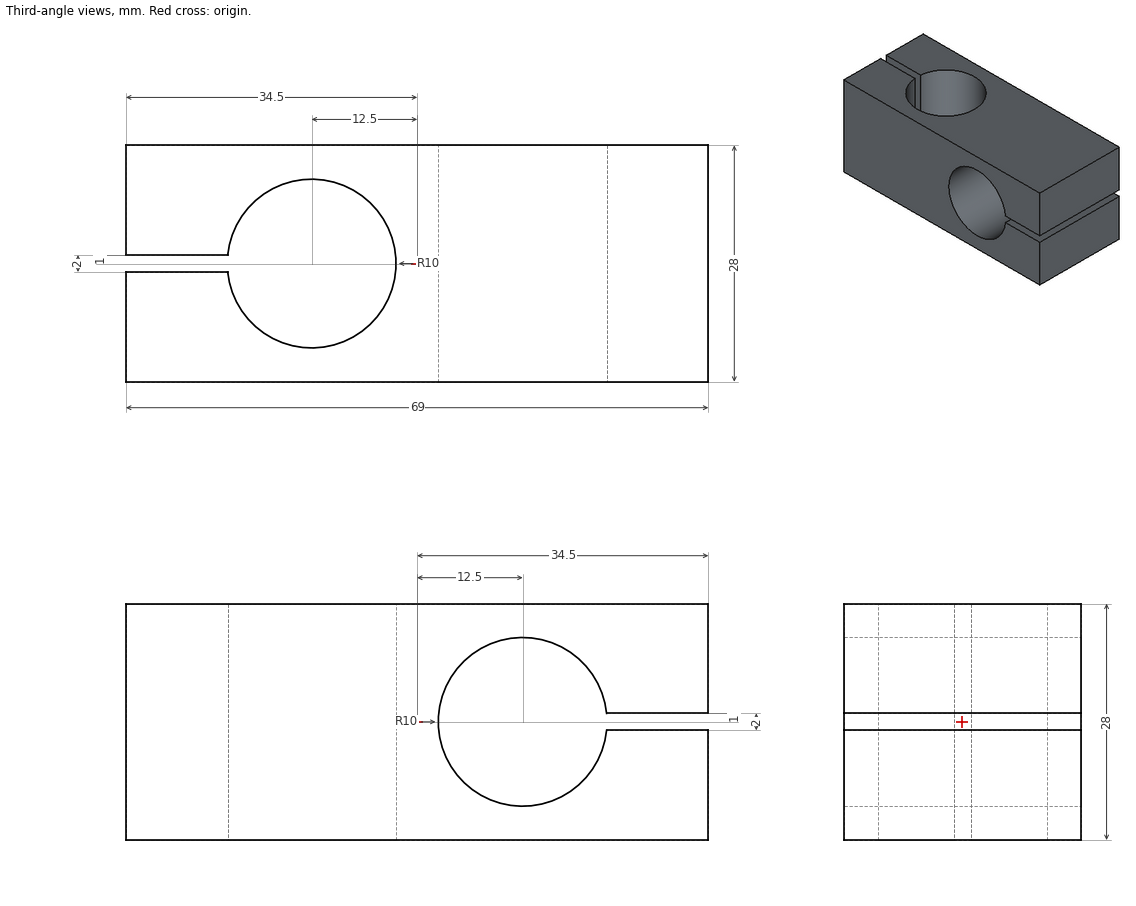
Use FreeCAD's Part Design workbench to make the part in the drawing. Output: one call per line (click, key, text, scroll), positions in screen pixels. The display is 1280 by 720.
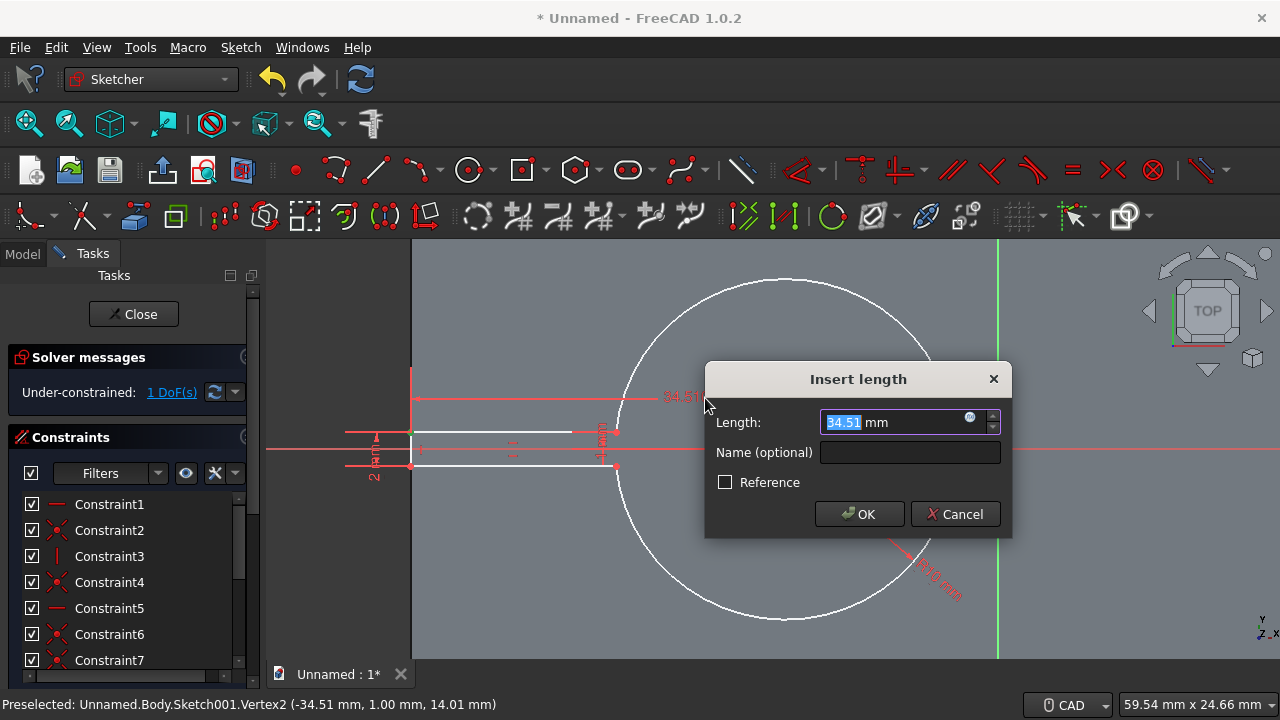
text(34.5)
key(Return)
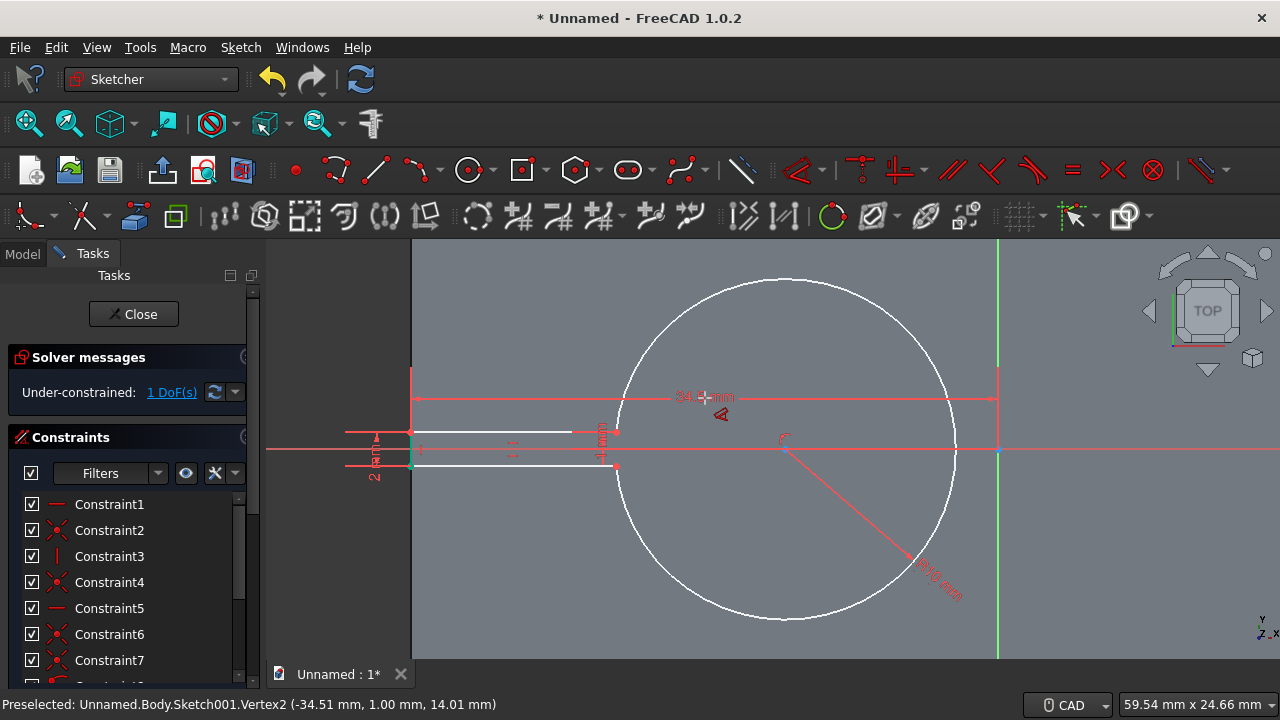
click(786, 449)
click(892, 483)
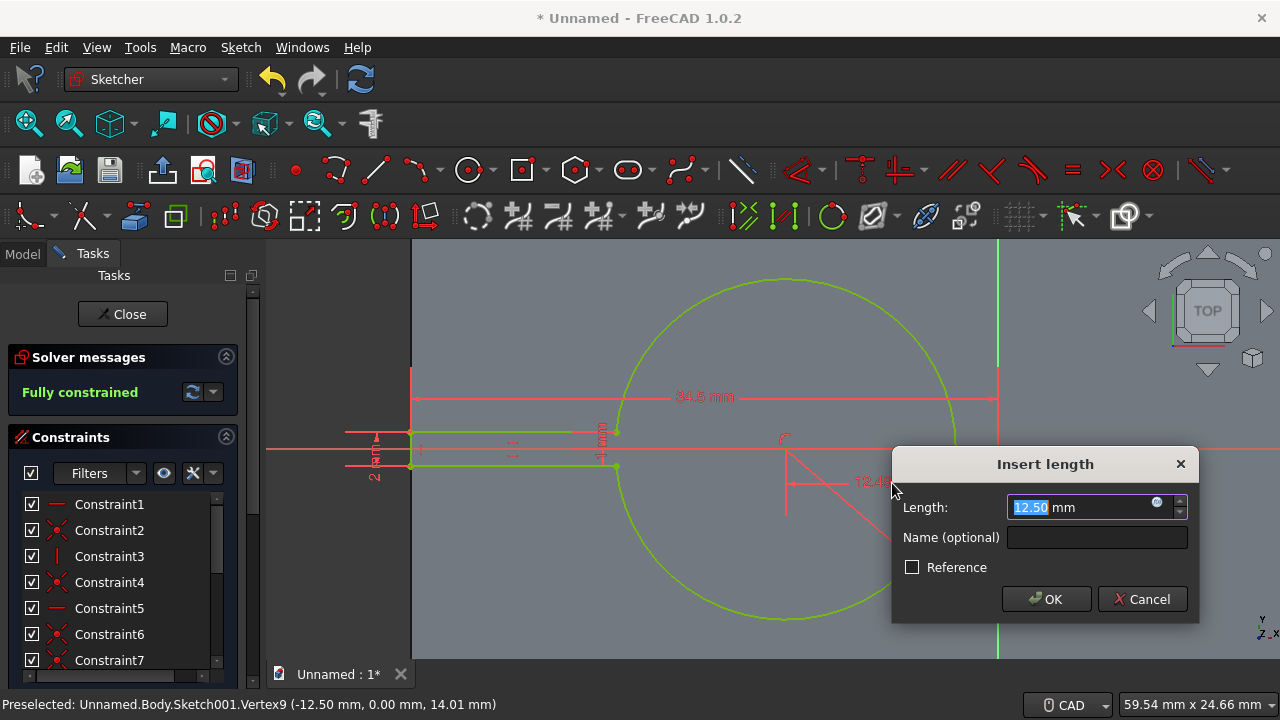
text(12.5)
key(Return)
key(Escape)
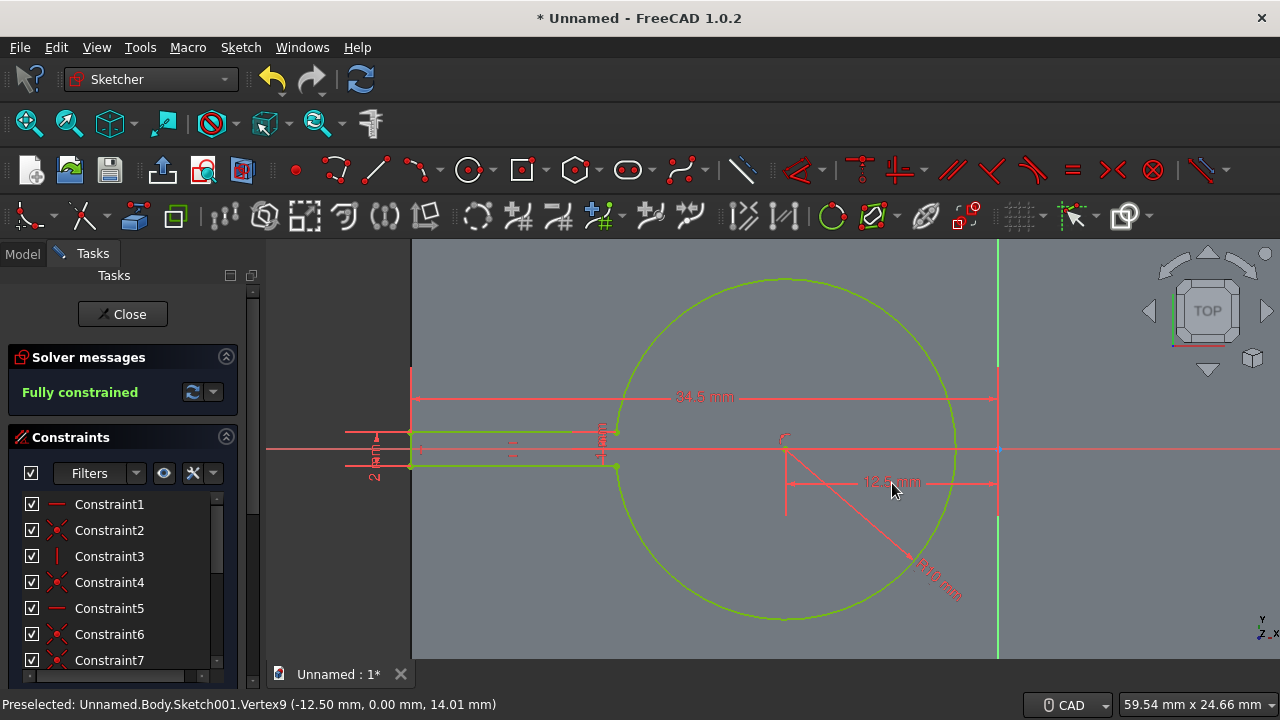
click(123, 314)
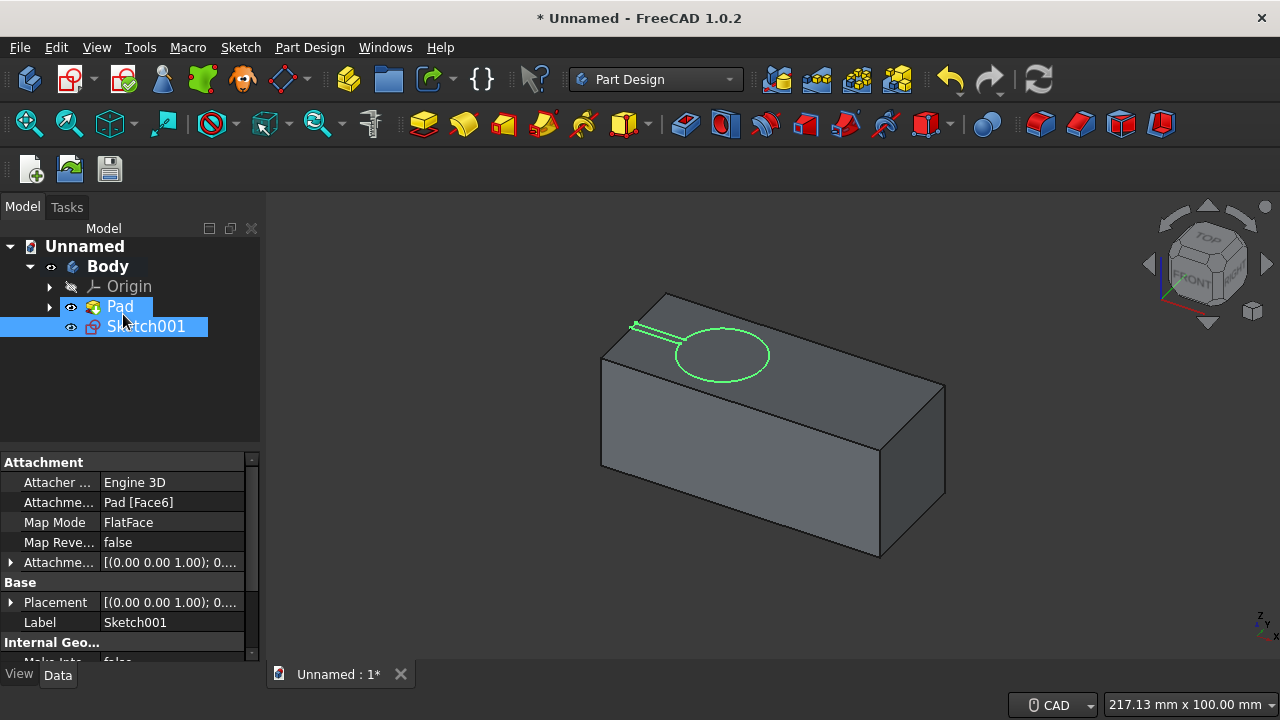
click(686, 124)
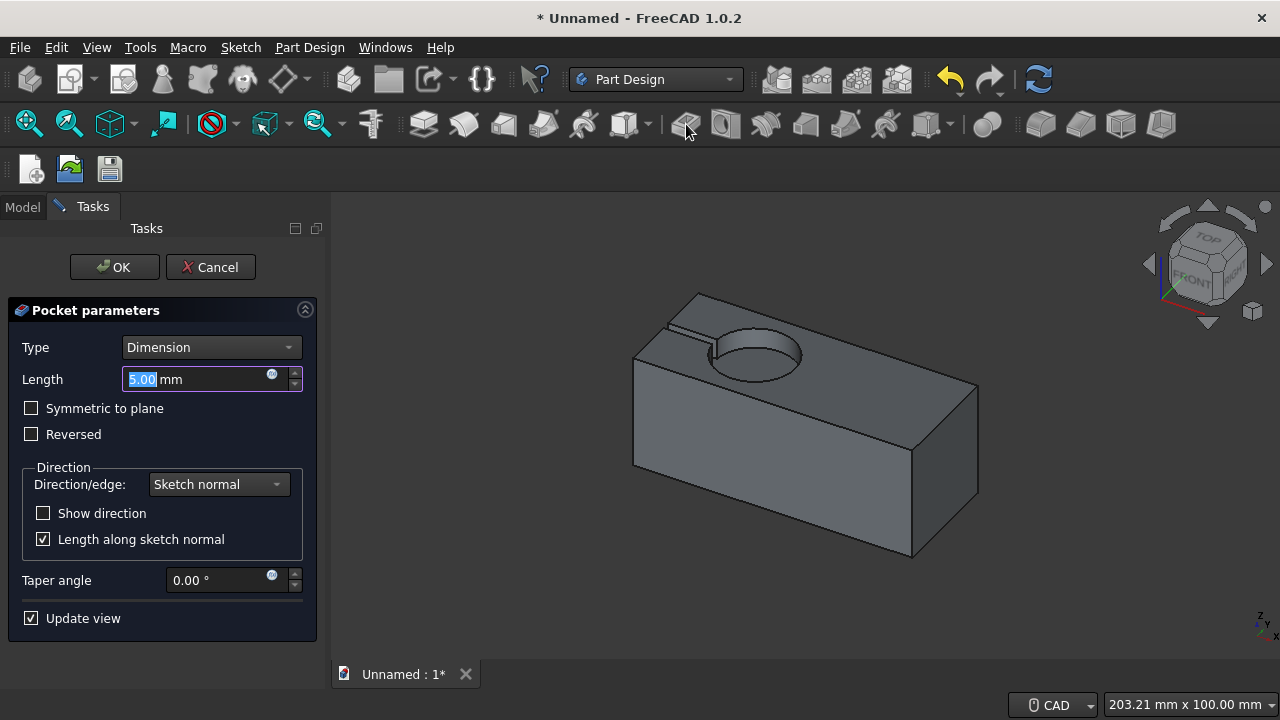
click(212, 348)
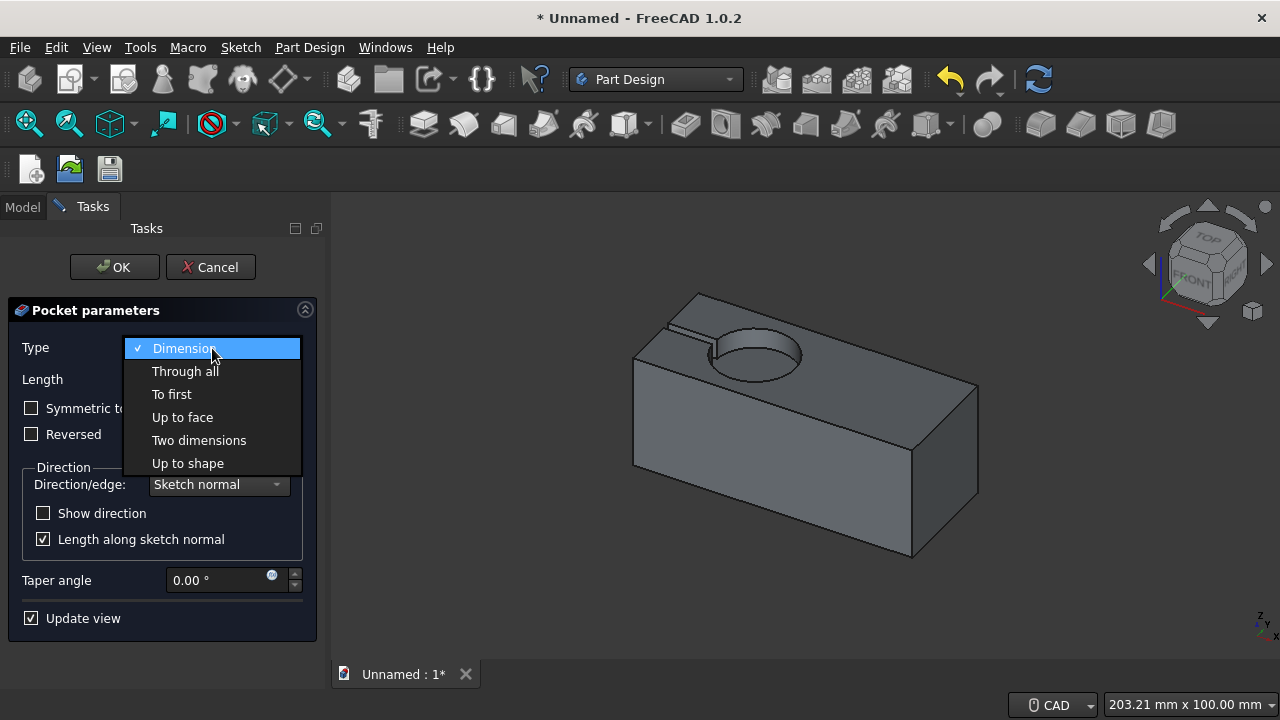
click(212, 372)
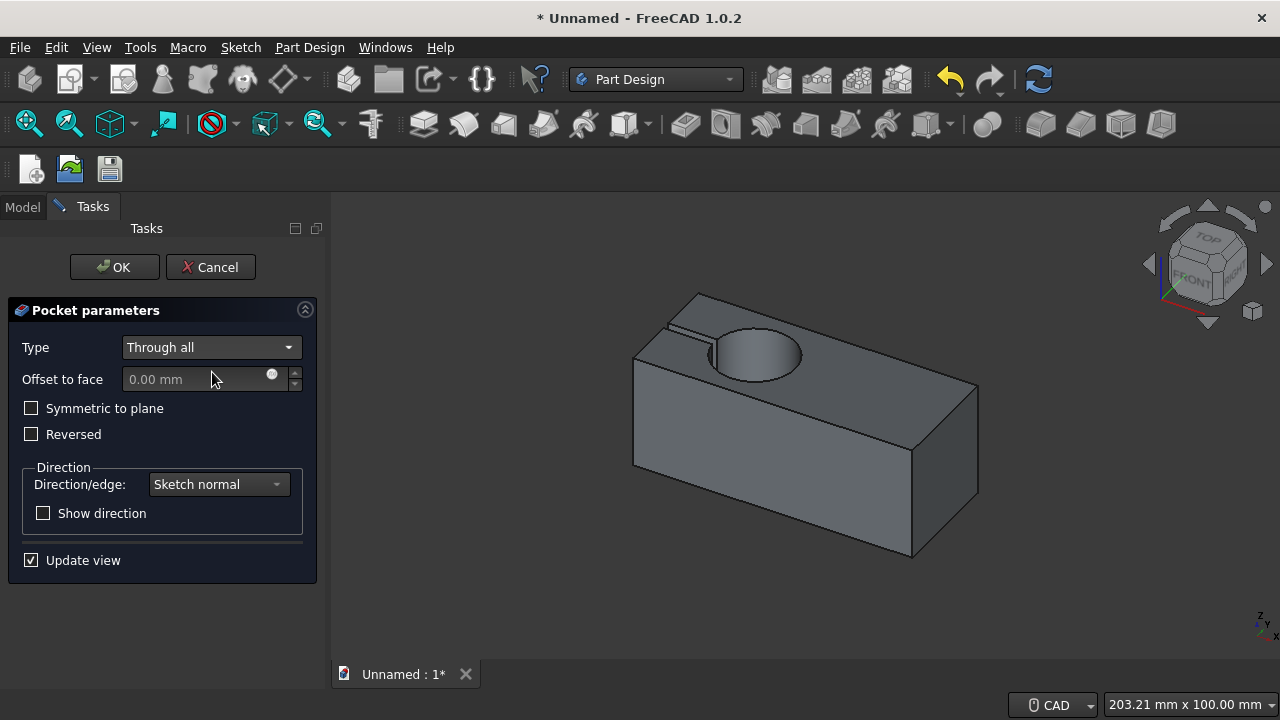
click(115, 267)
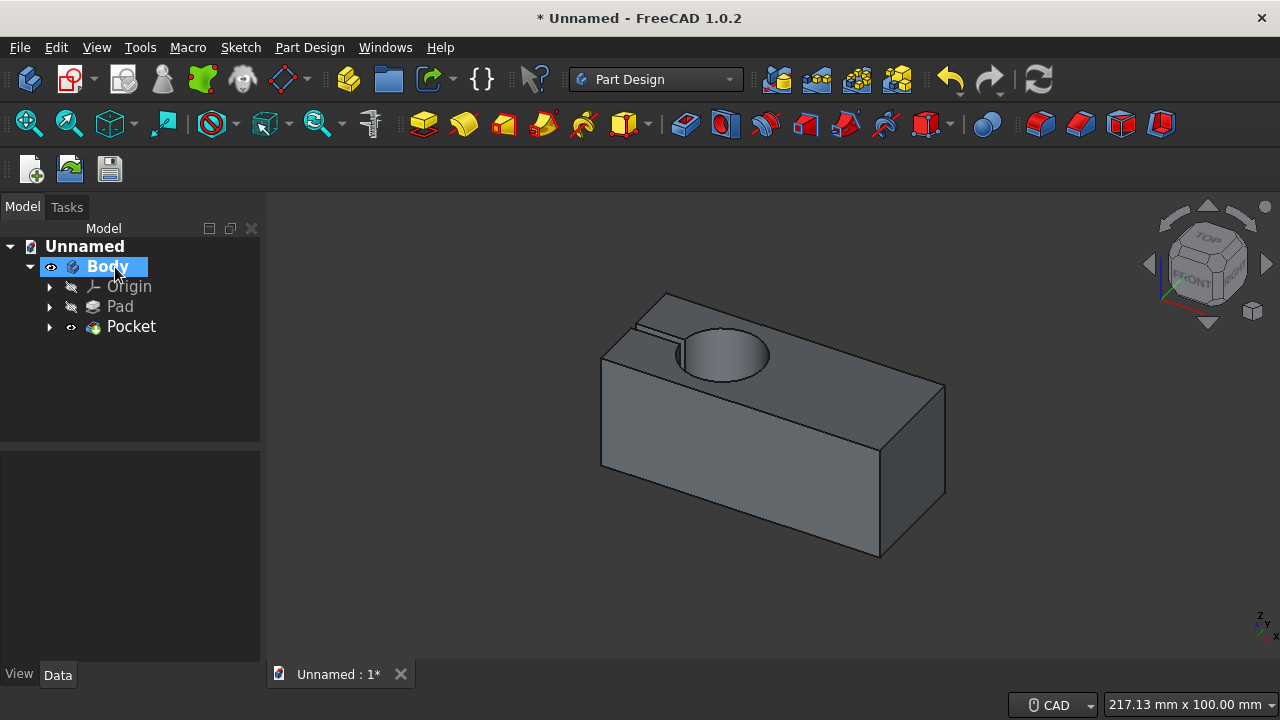
key(4)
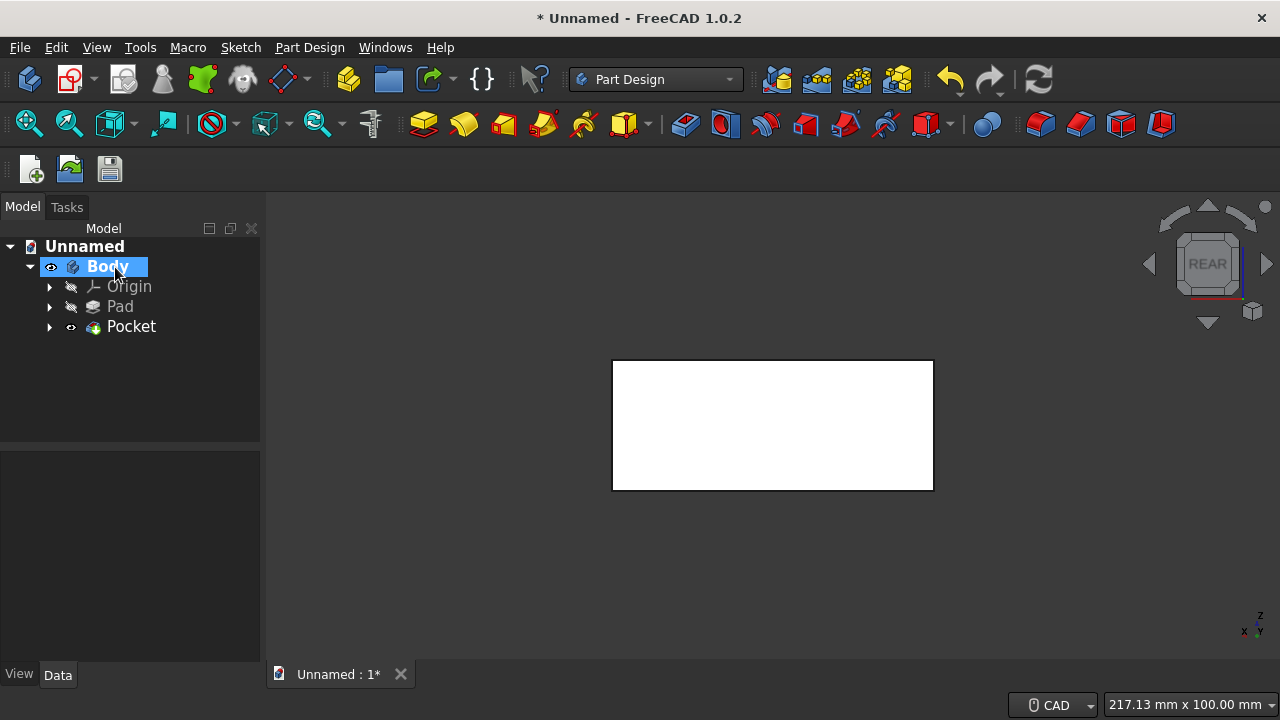
key(v)
key(f)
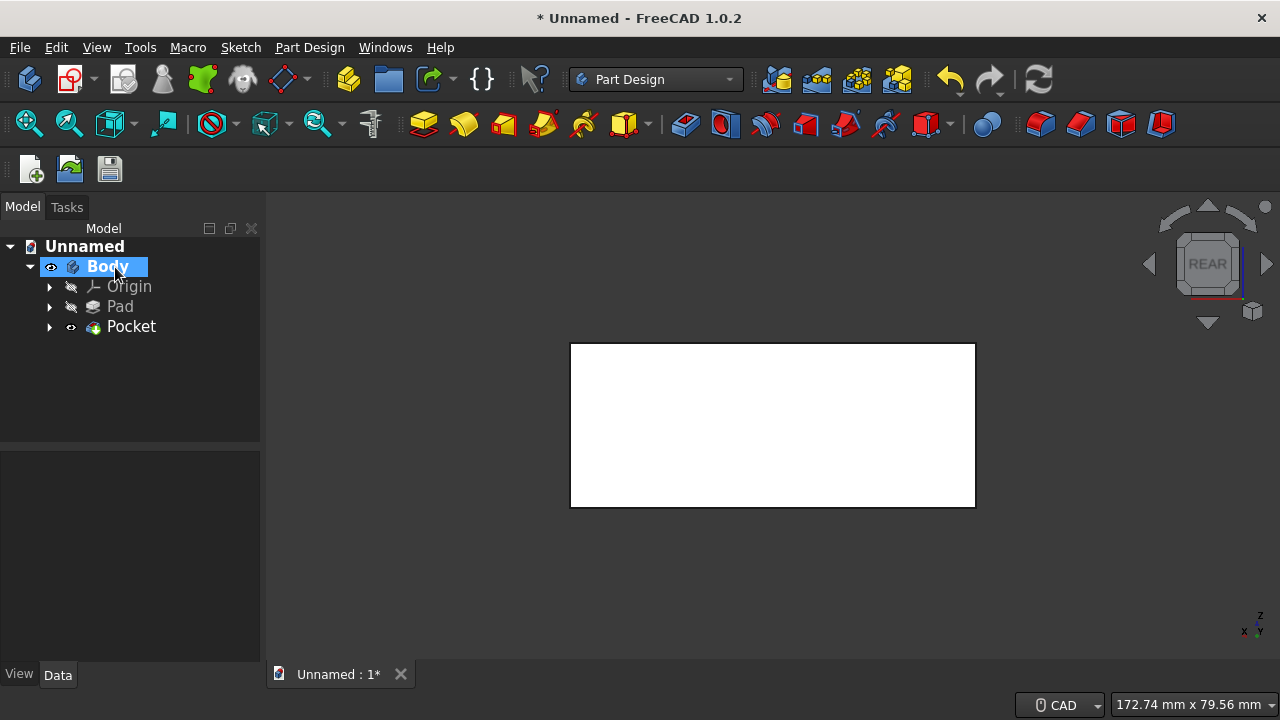
click(657, 425)